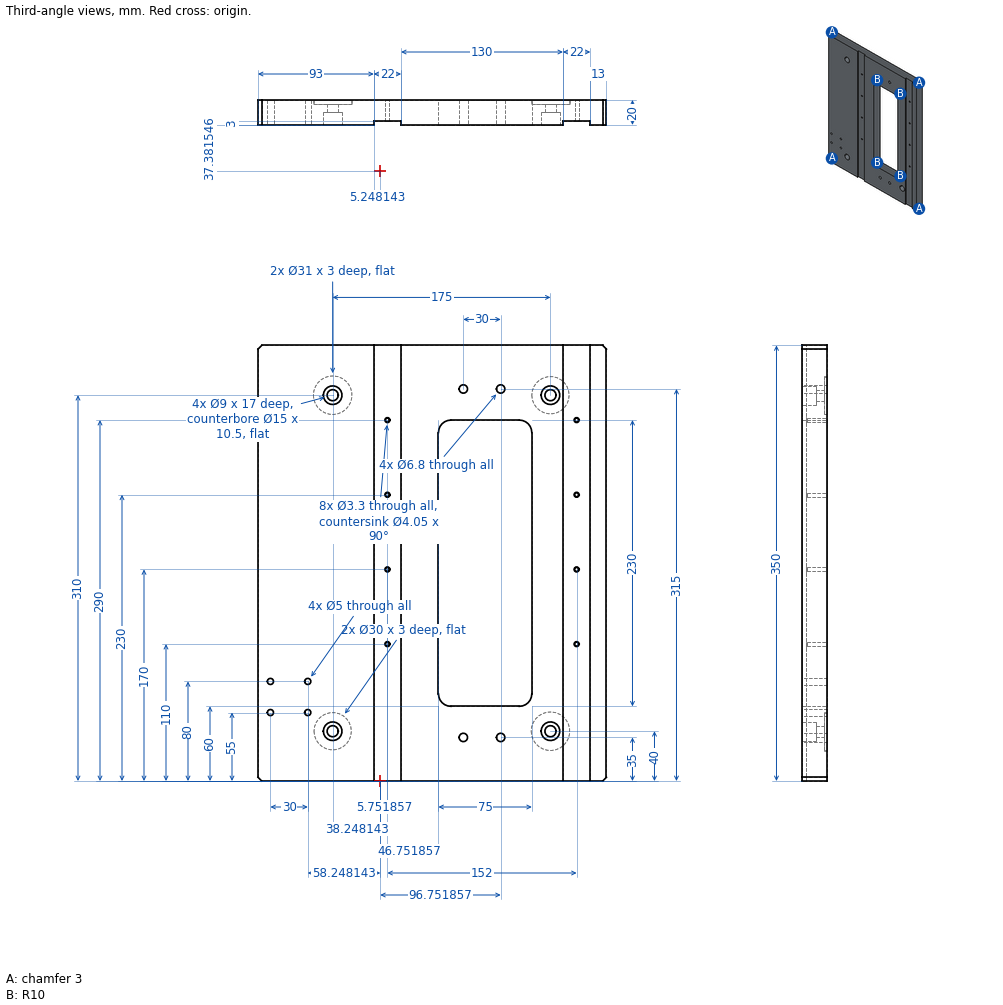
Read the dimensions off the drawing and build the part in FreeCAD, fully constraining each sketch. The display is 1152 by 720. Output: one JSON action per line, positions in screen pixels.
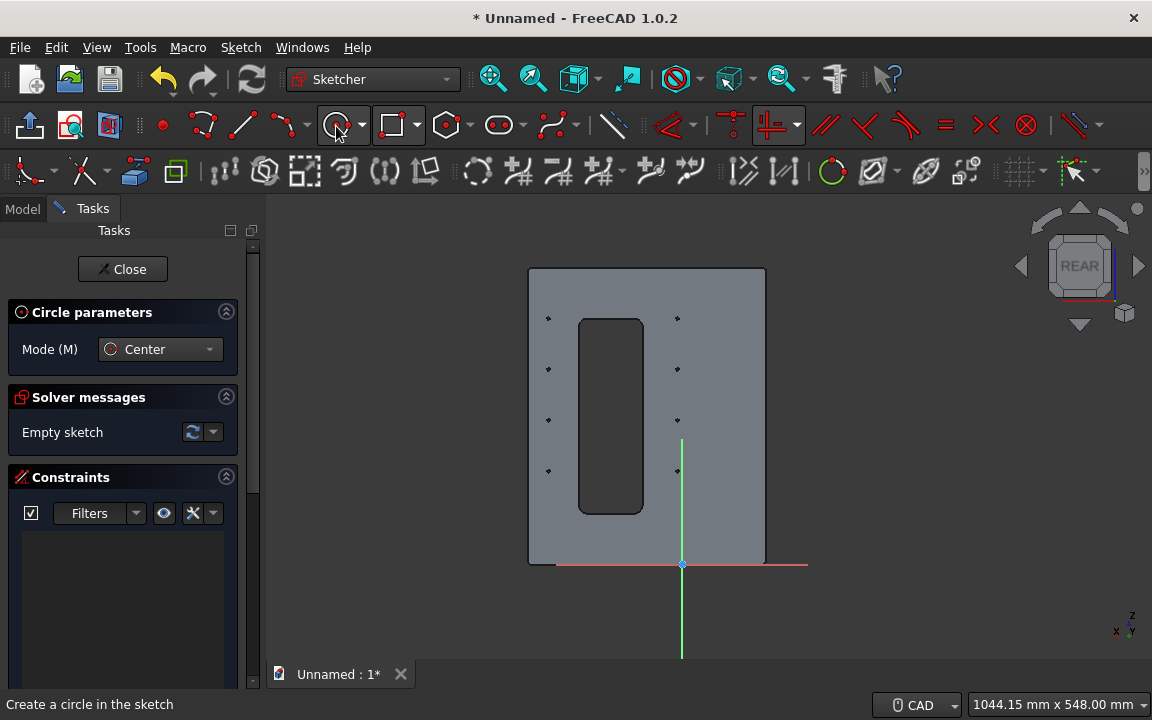
{"action": "scroll", "coordinate": [715, 302], "scroll_direction": "up", "scroll_amount": 3}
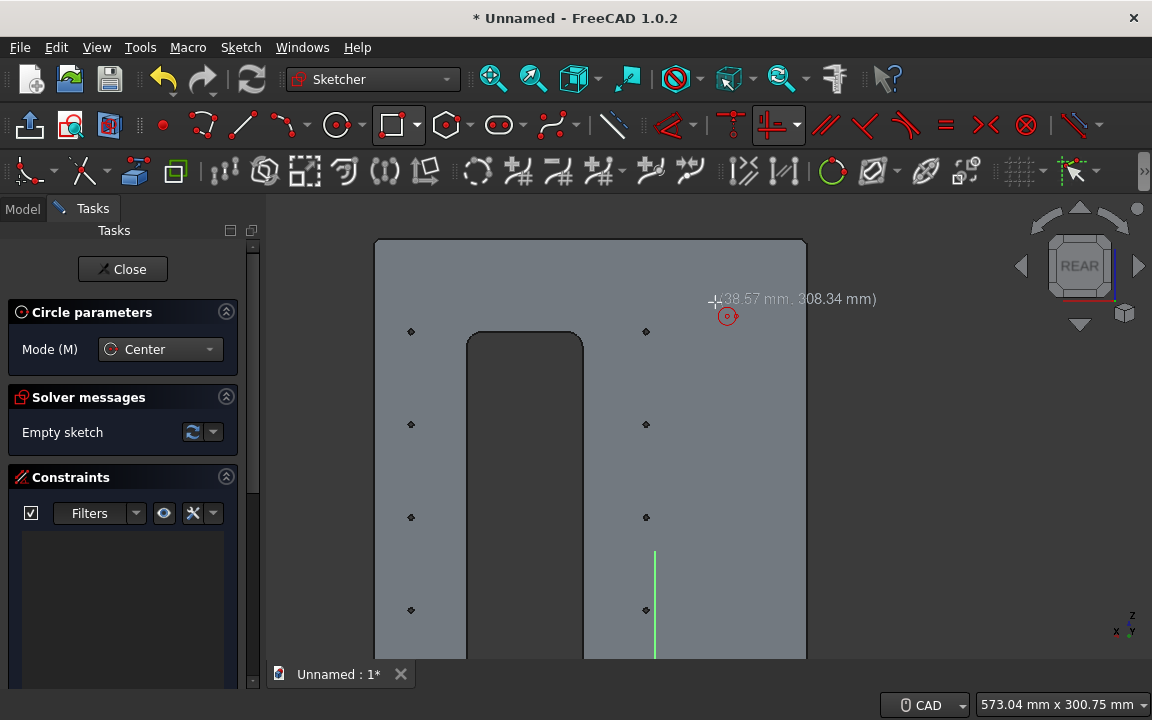
{"action": "left_click", "coordinate": [714, 301]}
{"action": "mouse_move", "coordinate": [731, 284]}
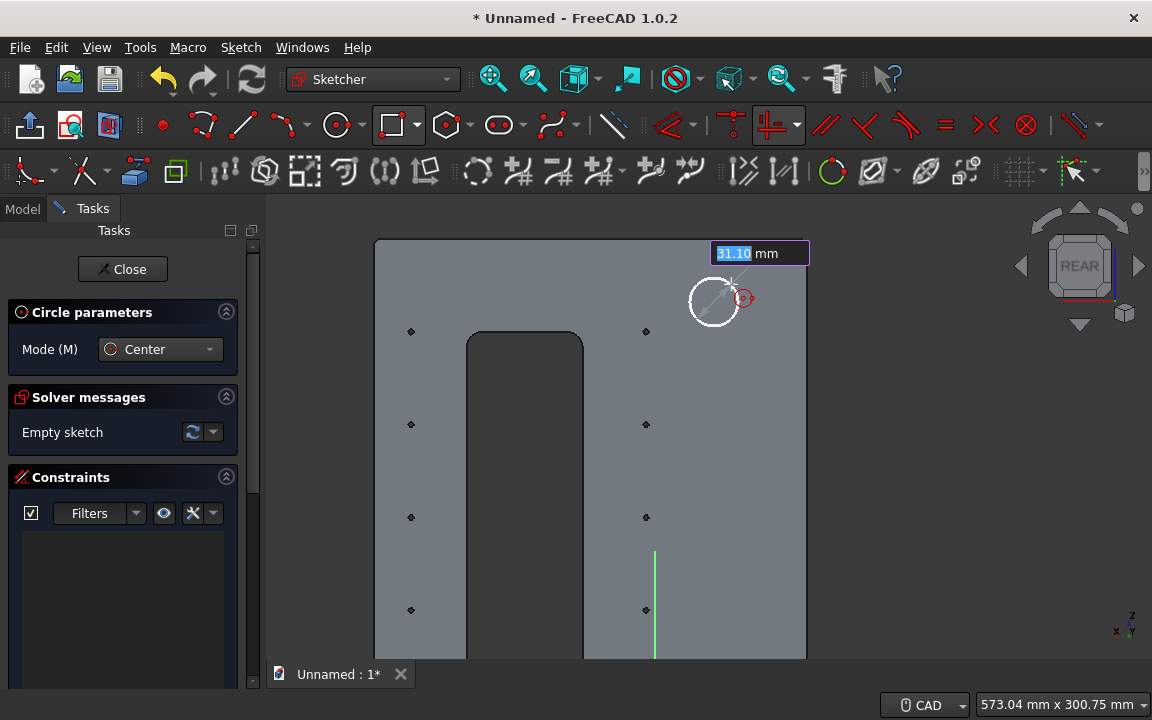
{"action": "type", "text": "31"}
{"action": "key", "text": "Return"}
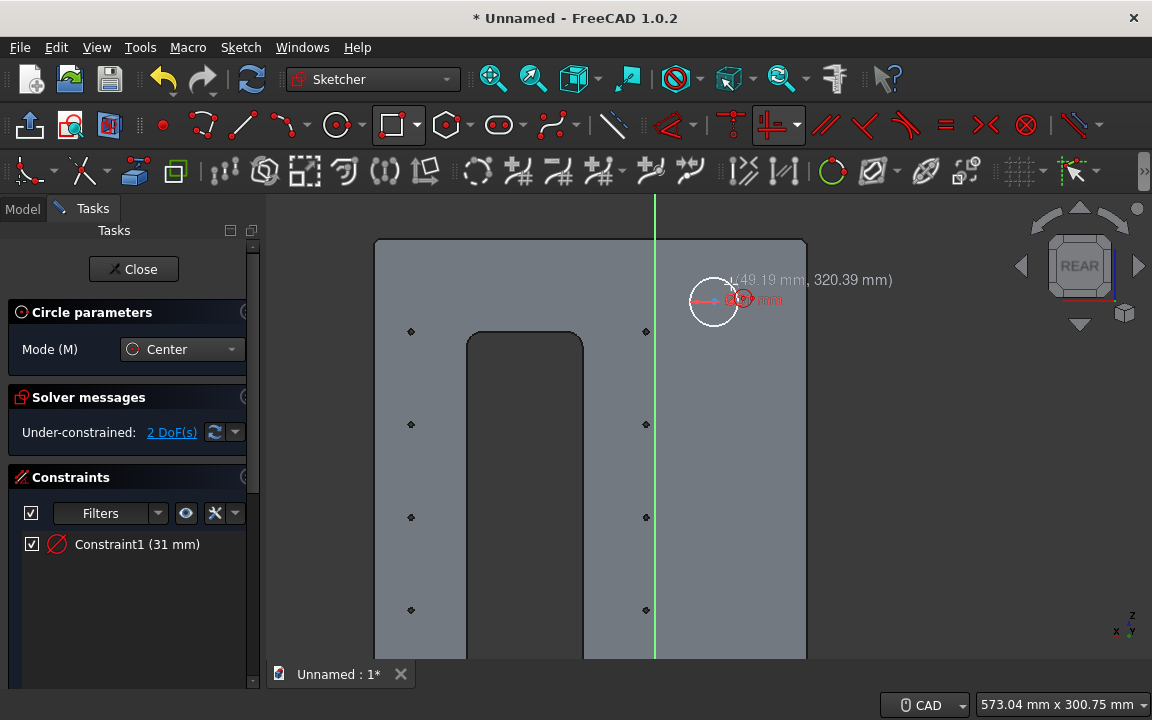
{"action": "scroll", "coordinate": [716, 302], "scroll_direction": "down", "scroll_amount": 3}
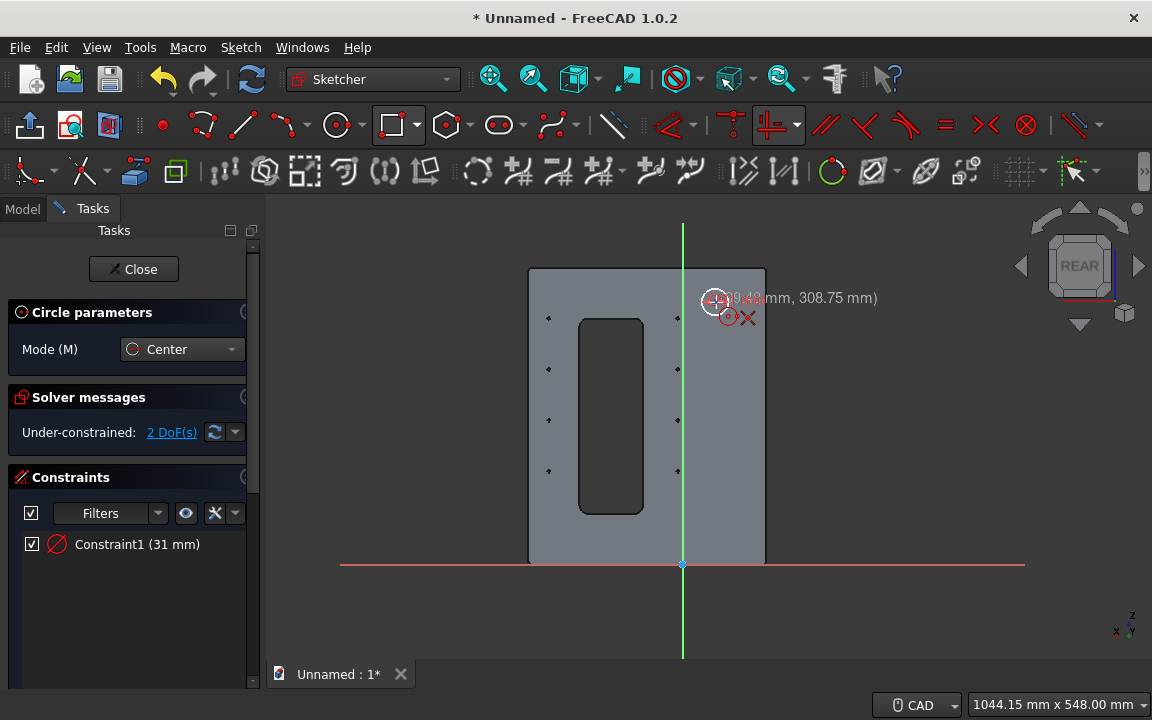
{"action": "scroll", "coordinate": [567, 531], "scroll_direction": "up", "scroll_amount": 3}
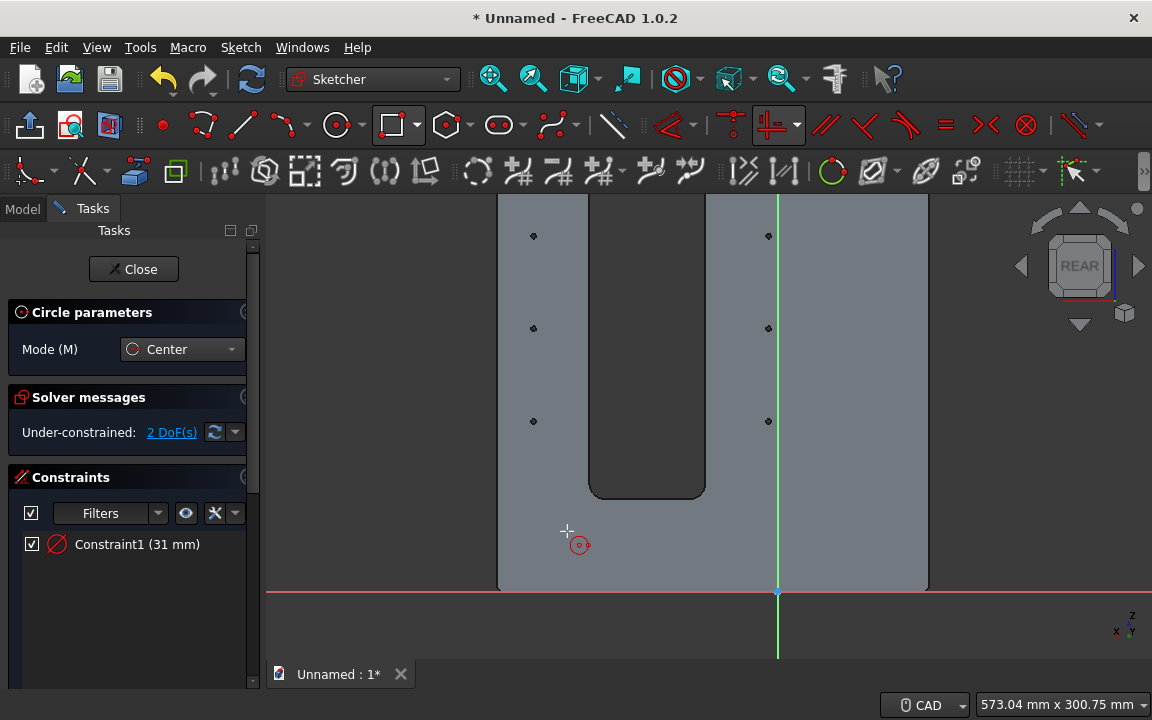
{"action": "left_click", "coordinate": [566, 530]}
{"action": "mouse_move", "coordinate": [583, 513]}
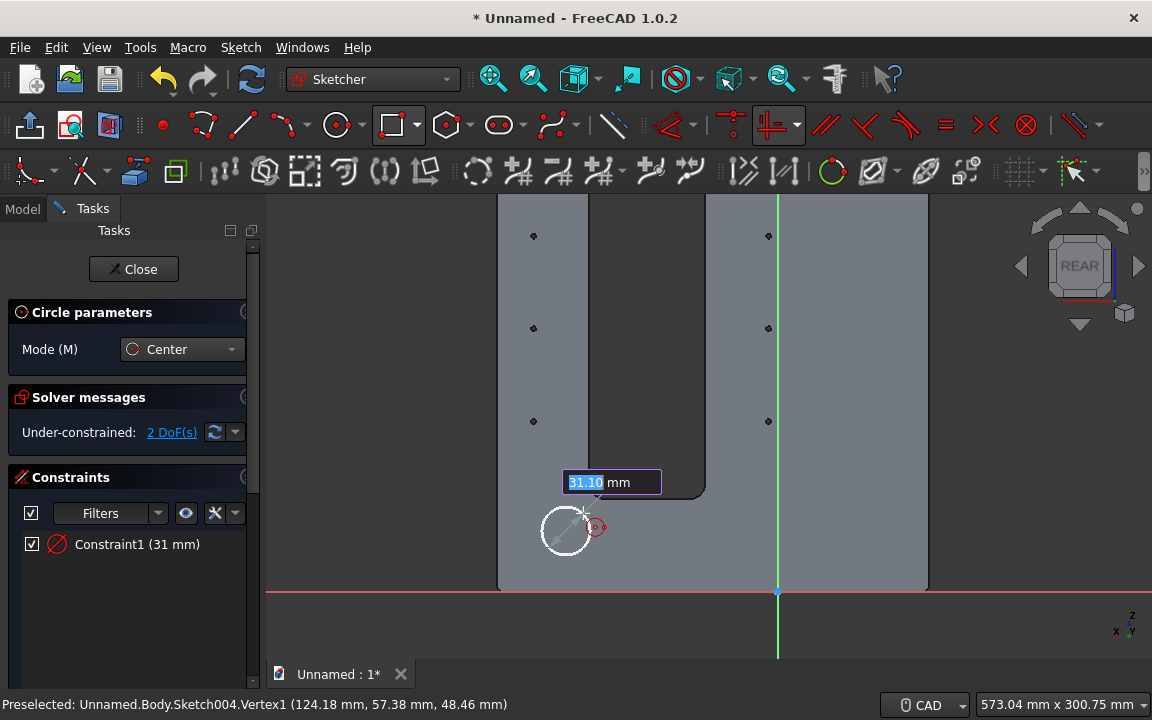
{"action": "type", "text": "31"}
{"action": "key", "text": "Return"}
{"action": "key", "text": "Escape"}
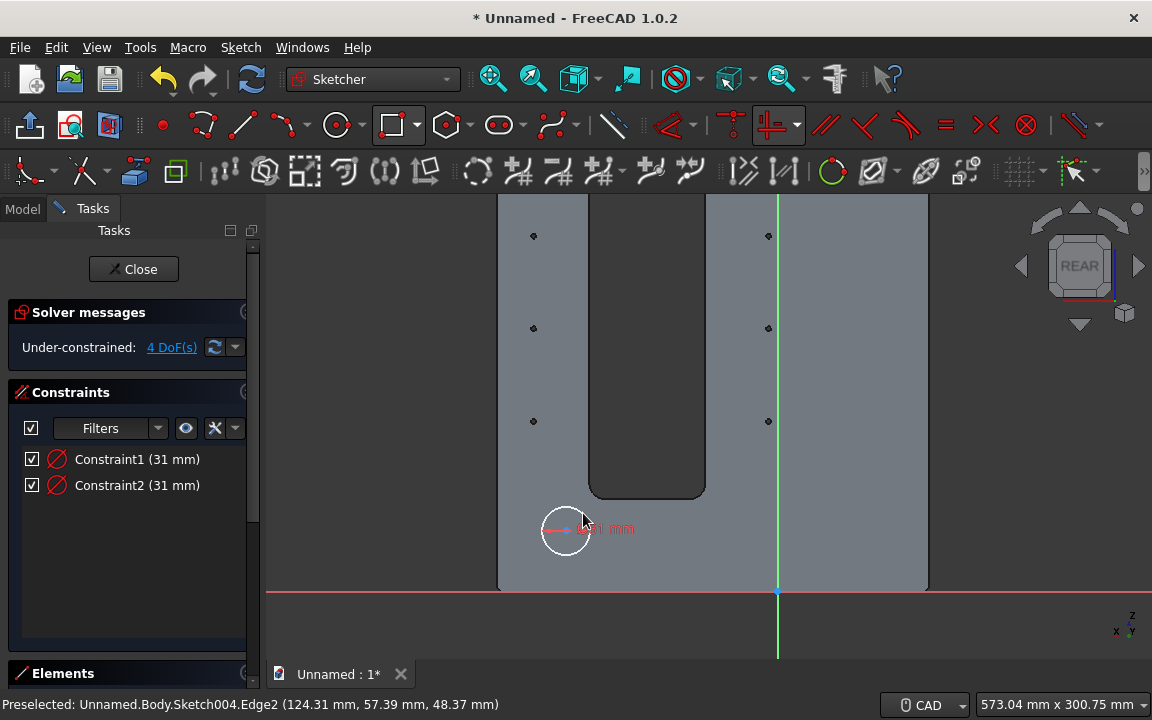
{"action": "left_click", "coordinate": [668, 126]}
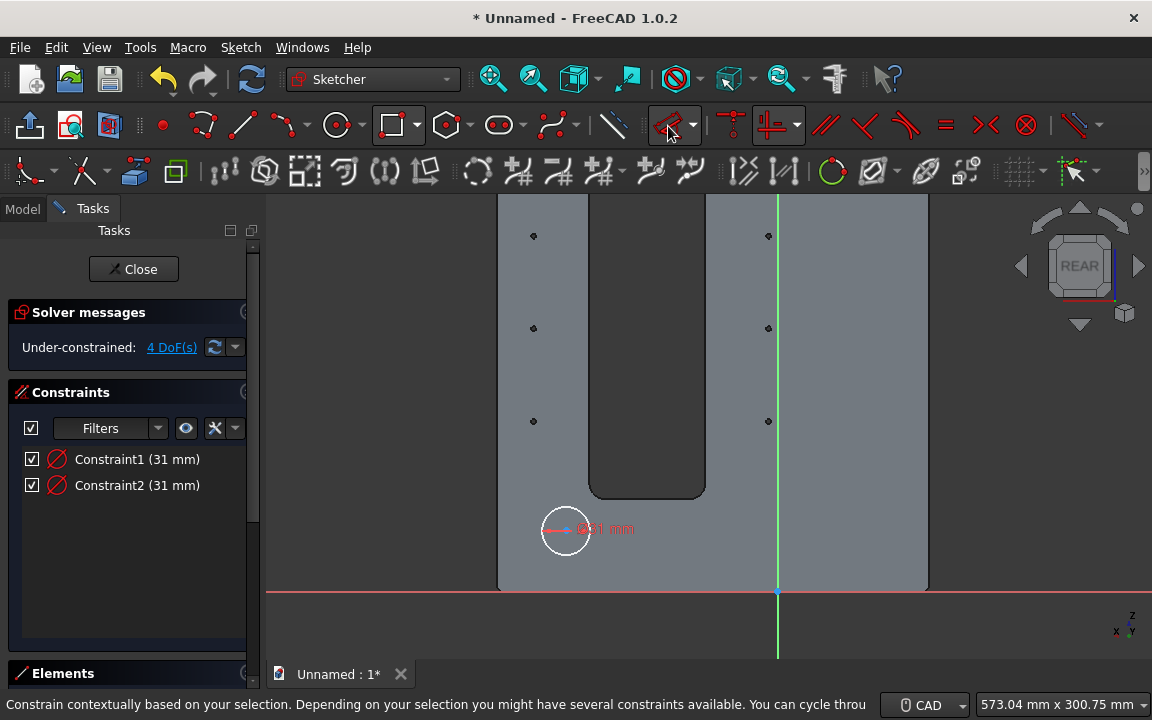
{"action": "left_click", "coordinate": [566, 531]}
{"action": "left_click", "coordinate": [532, 561]}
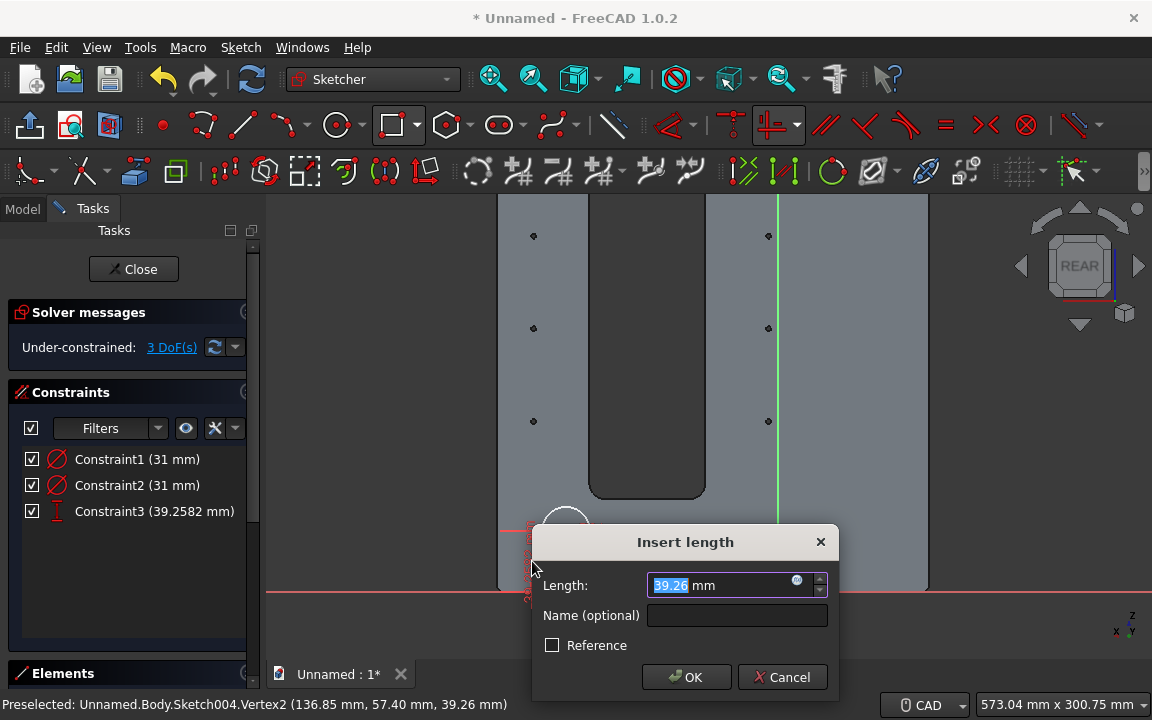
{"action": "type", "text": "40"}
{"action": "key", "text": "Return"}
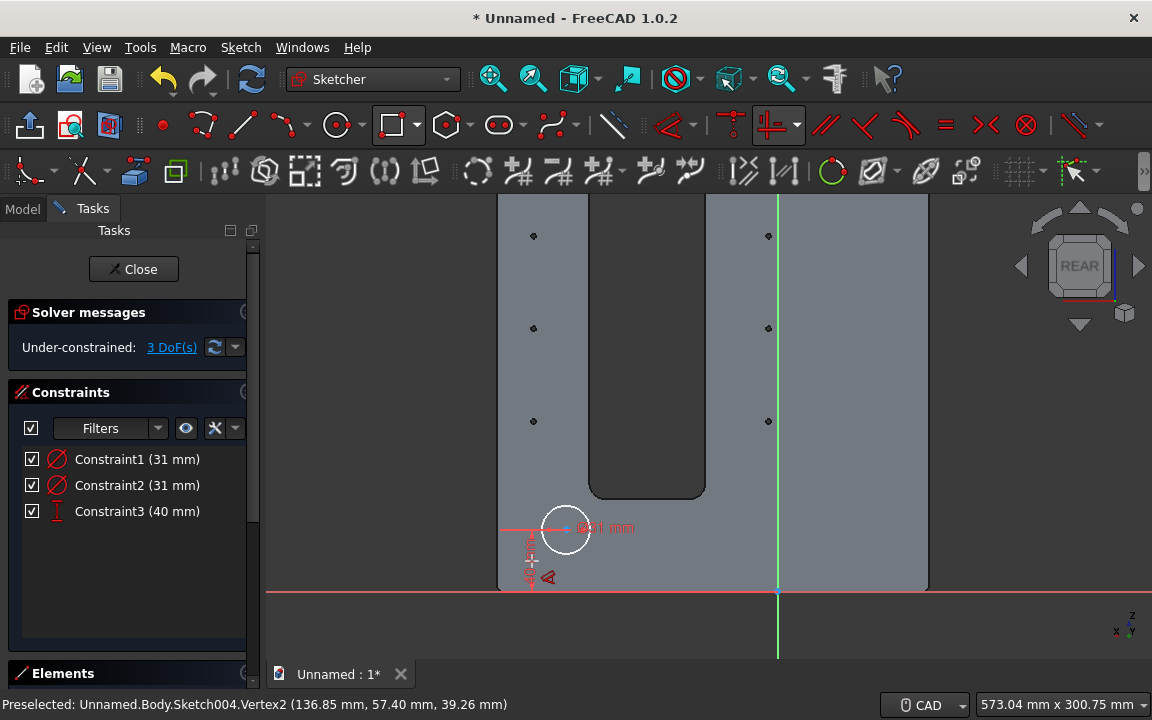
{"action": "scroll", "coordinate": [566, 532], "scroll_direction": "down", "scroll_amount": 3}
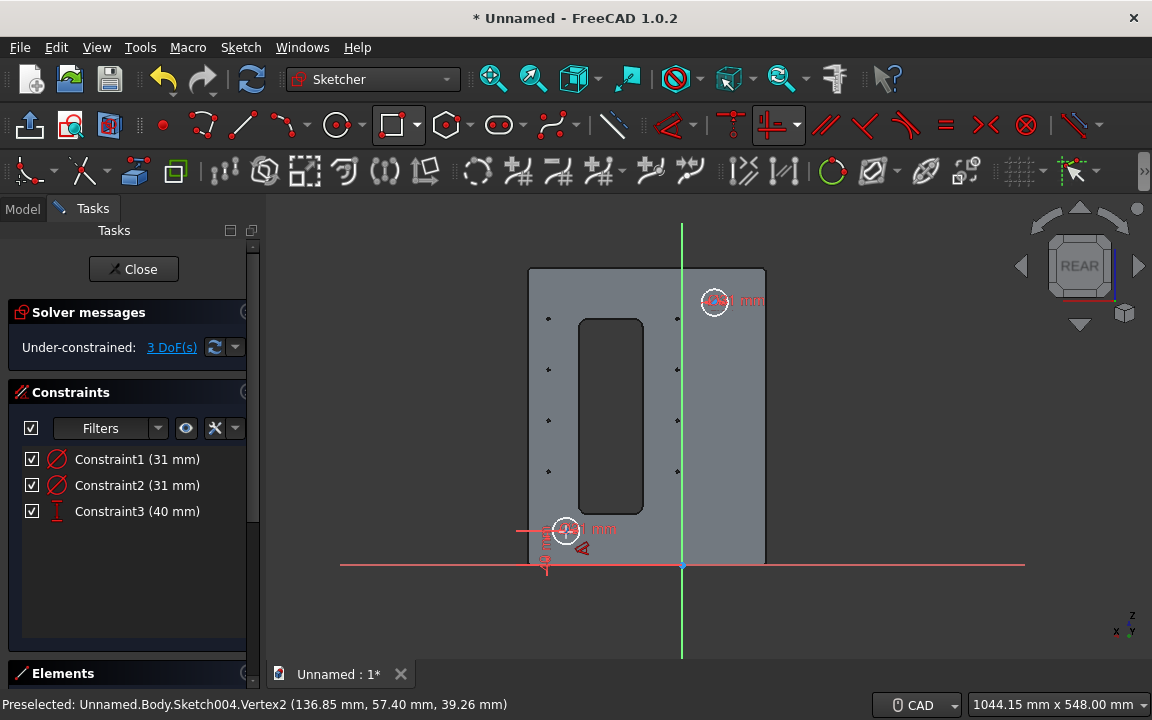
{"action": "left_click", "coordinate": [715, 303]}
{"action": "left_click", "coordinate": [749, 434]}